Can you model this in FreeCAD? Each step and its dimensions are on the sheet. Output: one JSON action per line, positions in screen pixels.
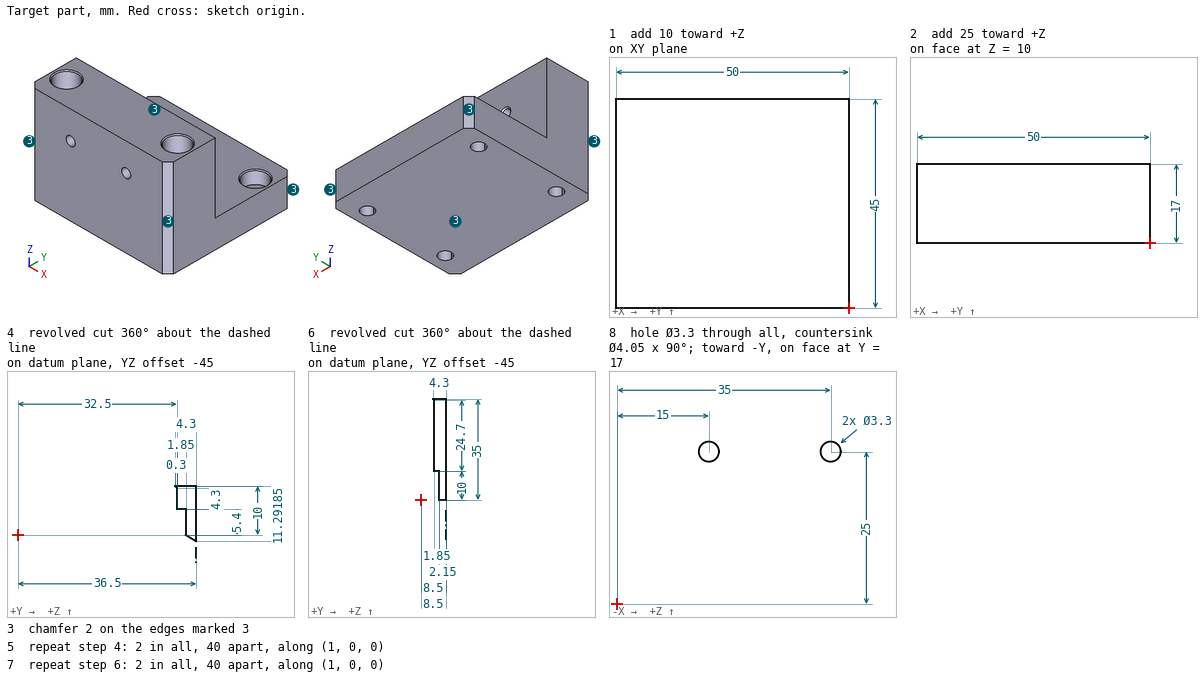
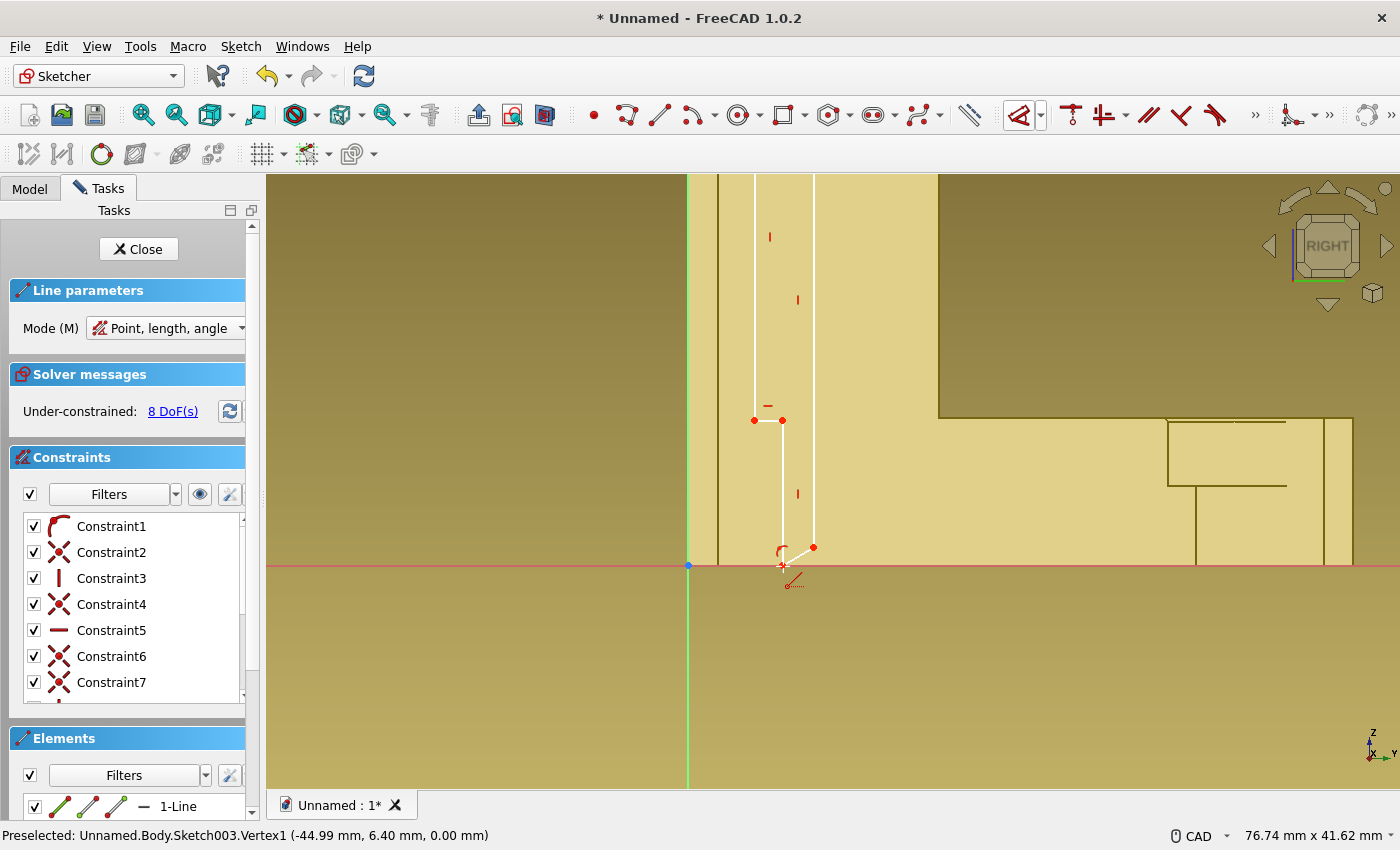
{"action": "left_click", "coordinate": [814, 618]}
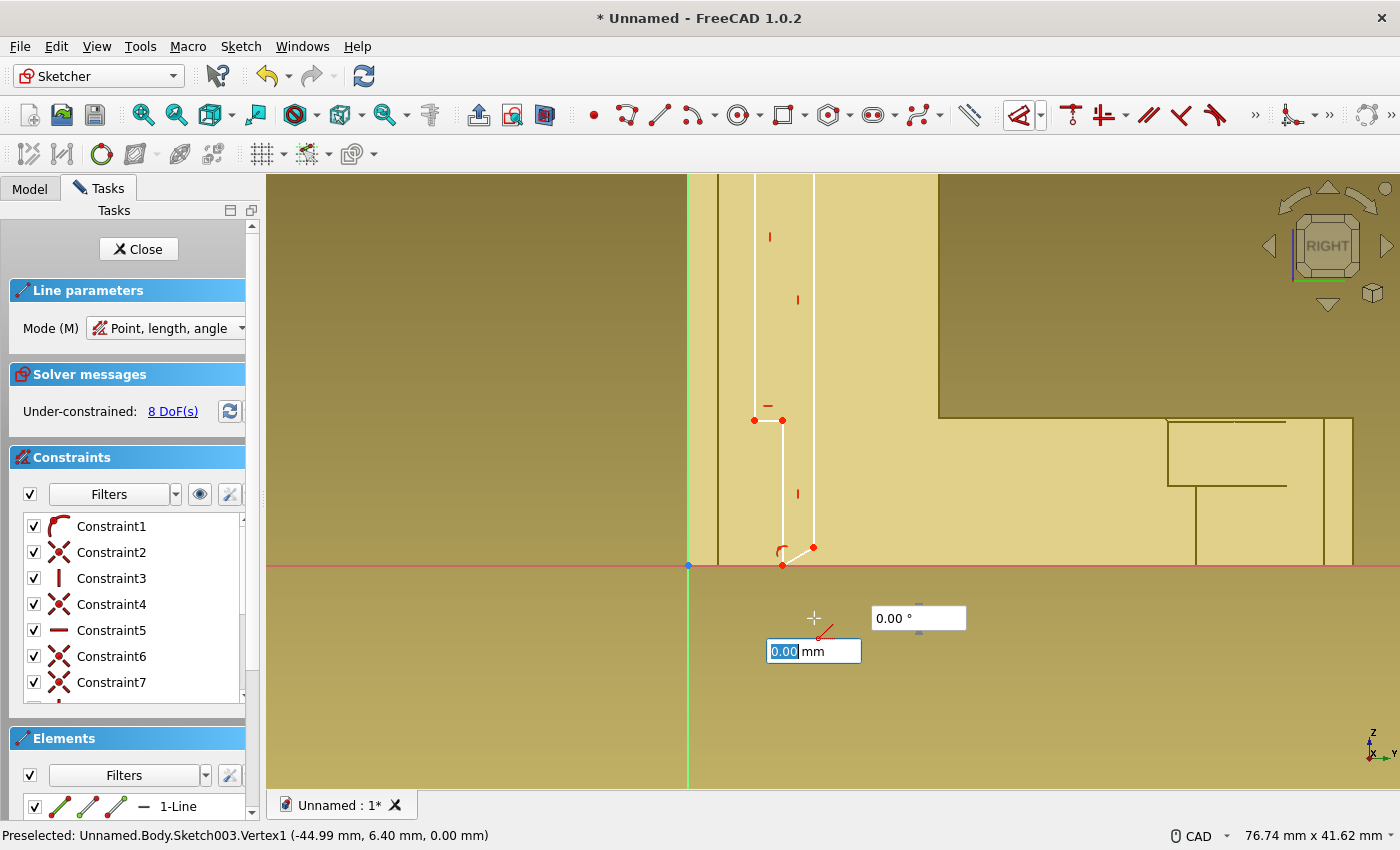
{"action": "scroll", "coordinate": [781, 568], "scroll_direction": "down", "scroll_amount": 3}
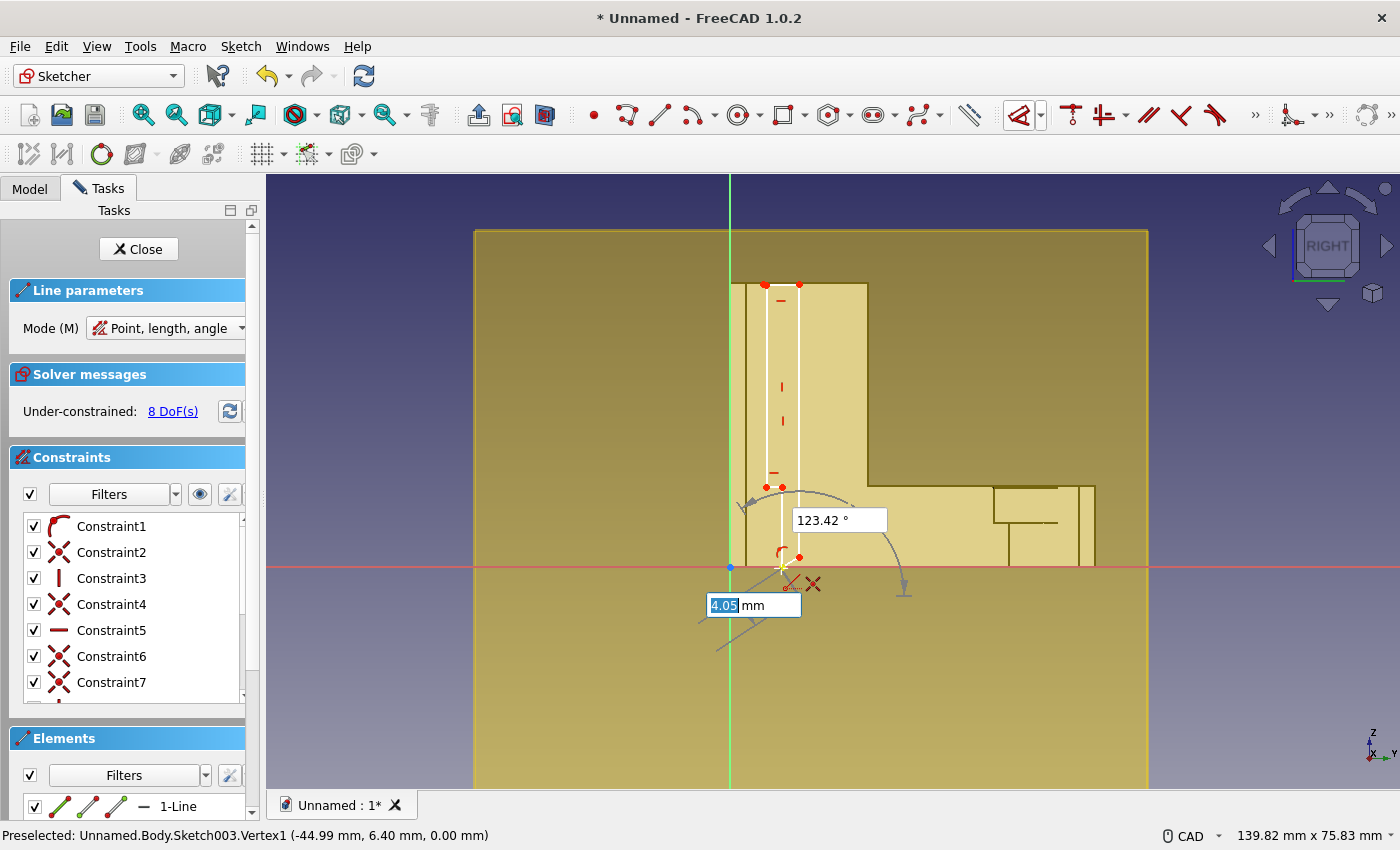
{"action": "left_click", "coordinate": [799, 681]}
{"action": "key", "text": "Escape"}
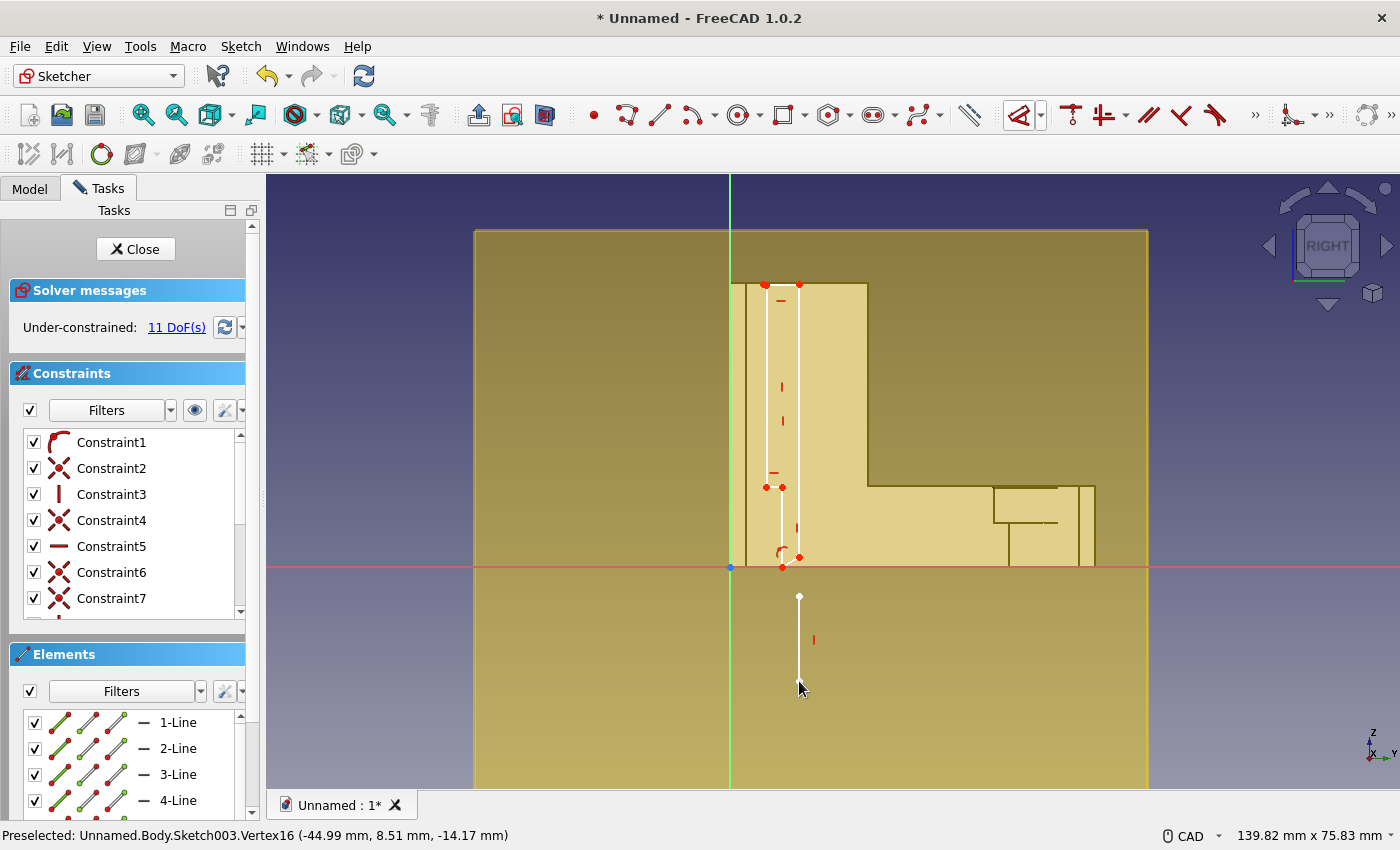
{"action": "left_click", "coordinate": [799, 622]}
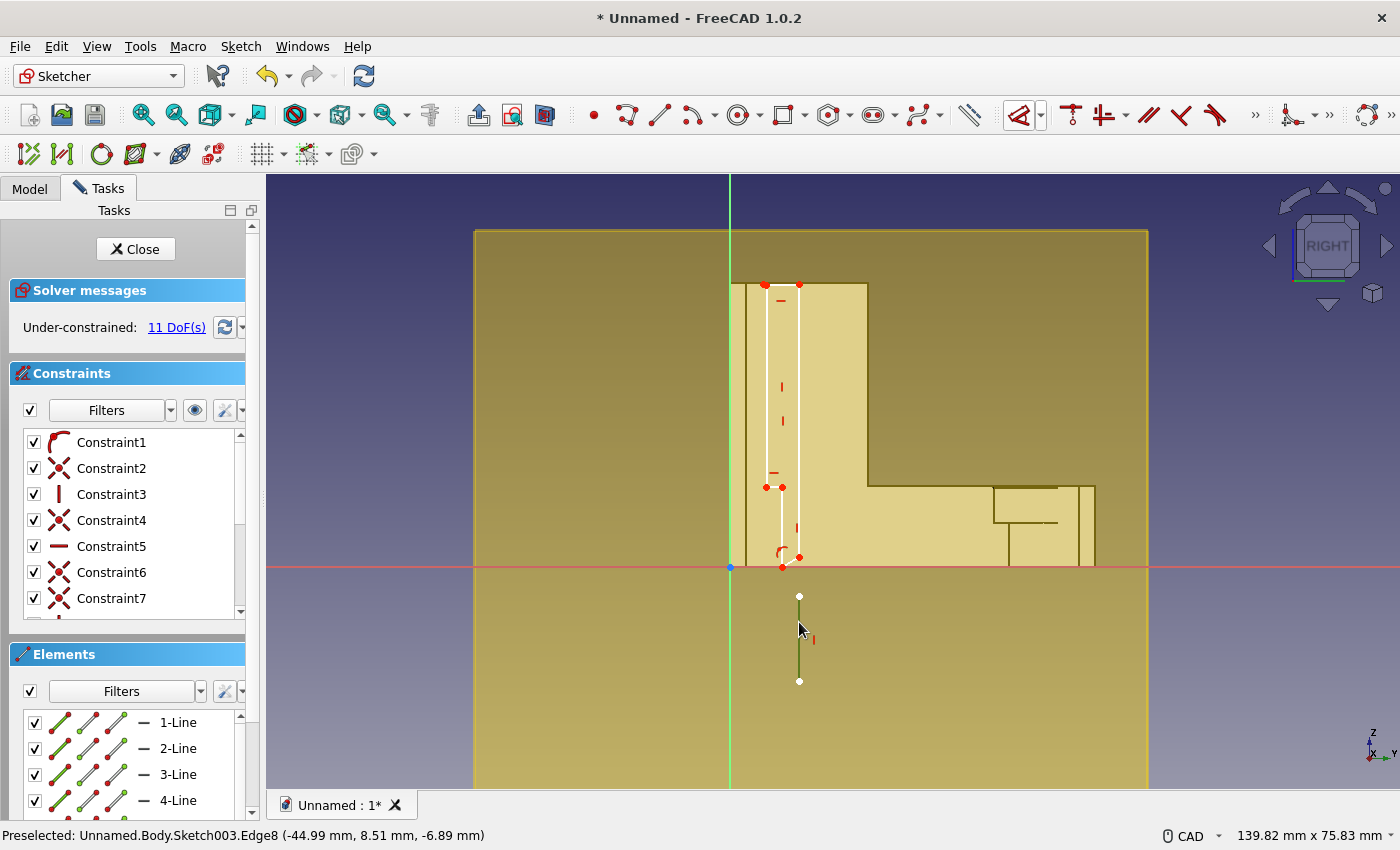
{"action": "left_click", "coordinate": [970, 116]}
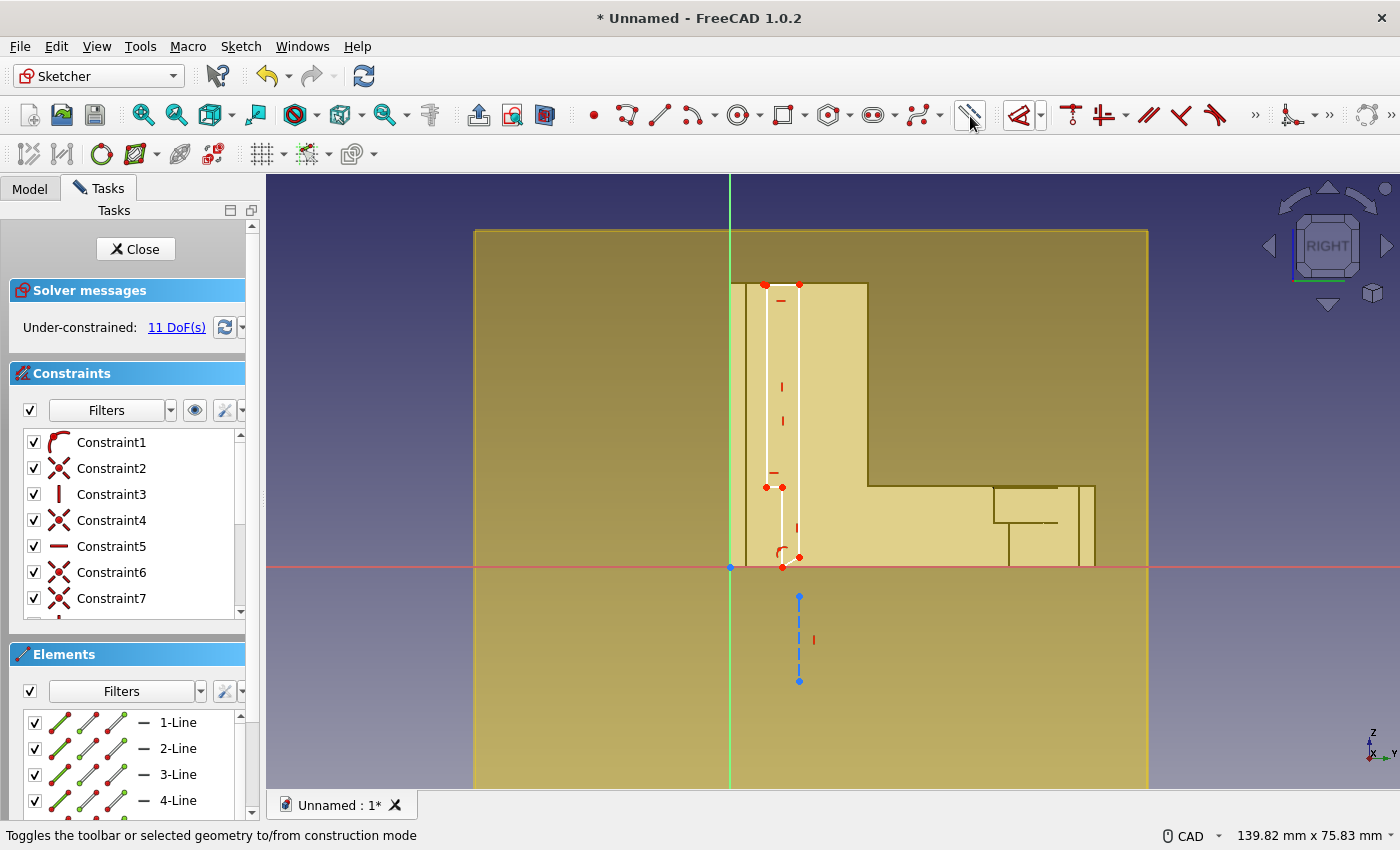
{"action": "scroll", "coordinate": [792, 561], "scroll_direction": "up", "scroll_amount": 5}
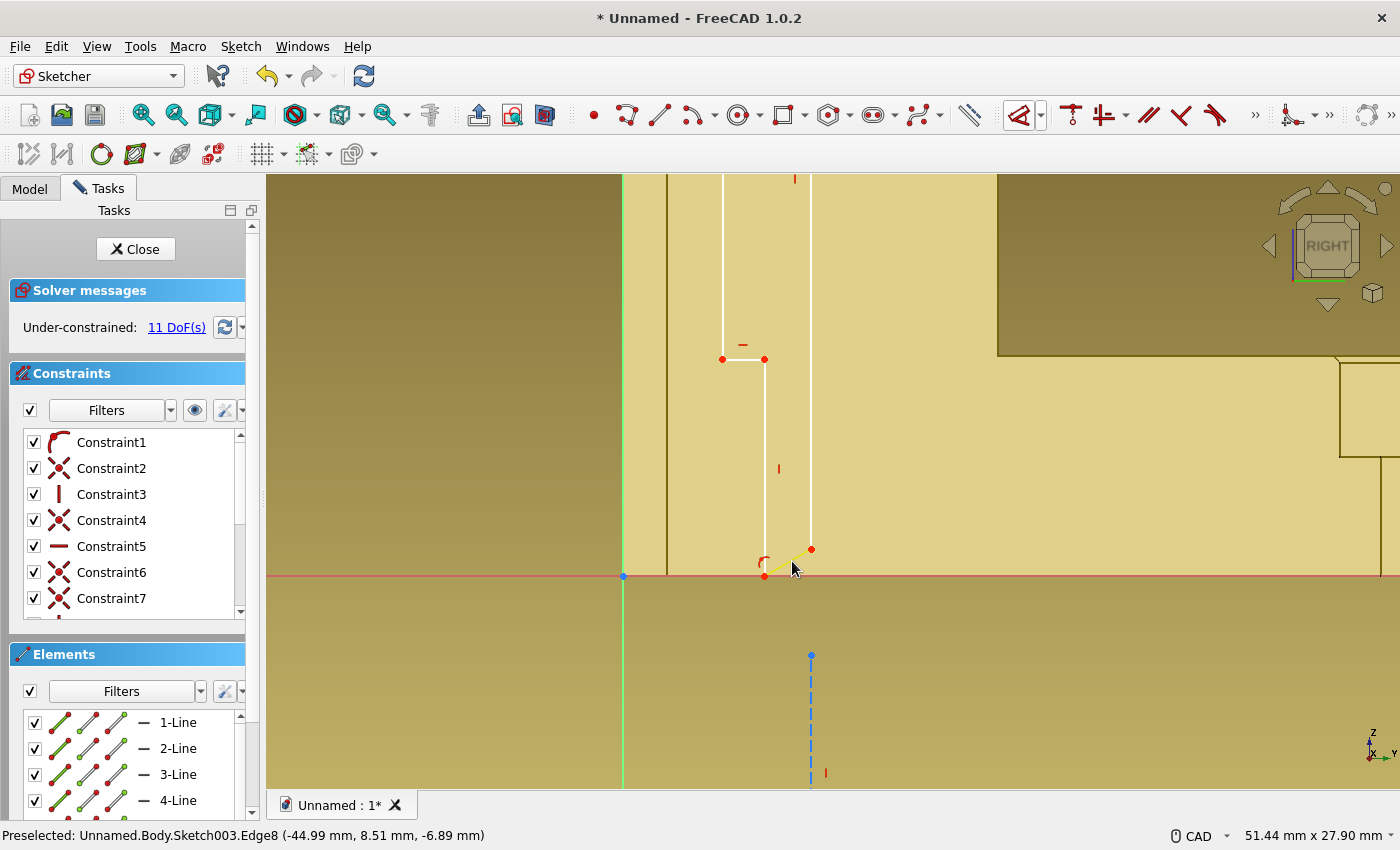
{"action": "left_click", "coordinate": [792, 560]}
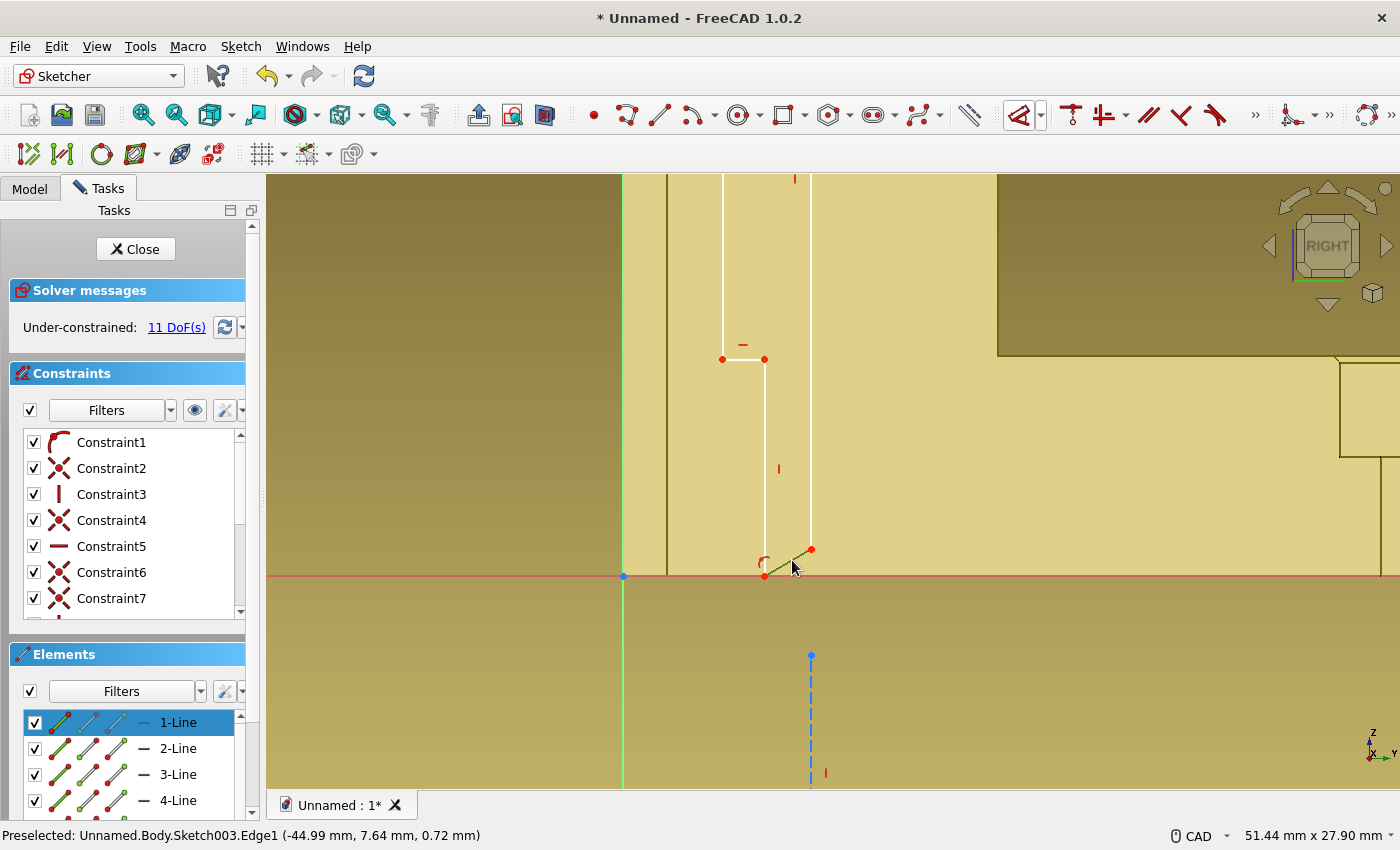
{"action": "key", "text": "h"}